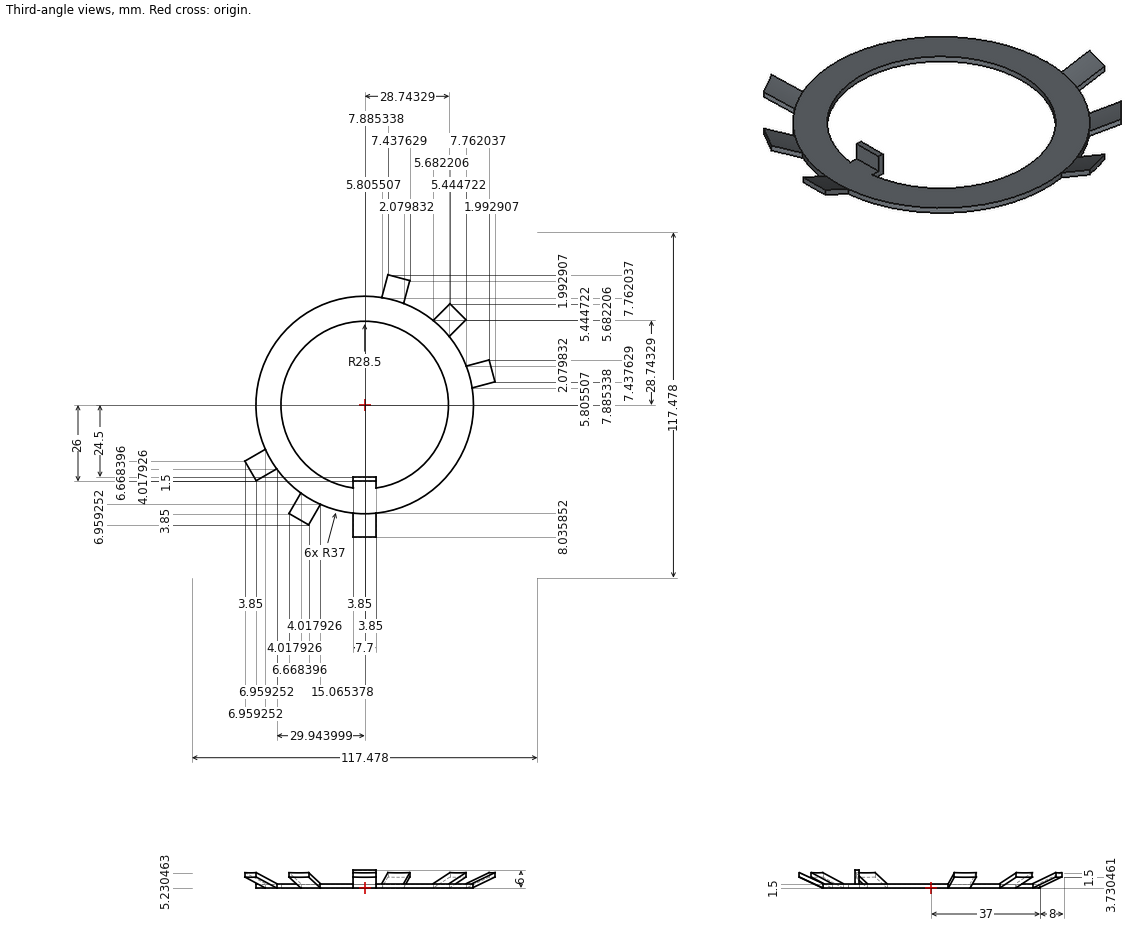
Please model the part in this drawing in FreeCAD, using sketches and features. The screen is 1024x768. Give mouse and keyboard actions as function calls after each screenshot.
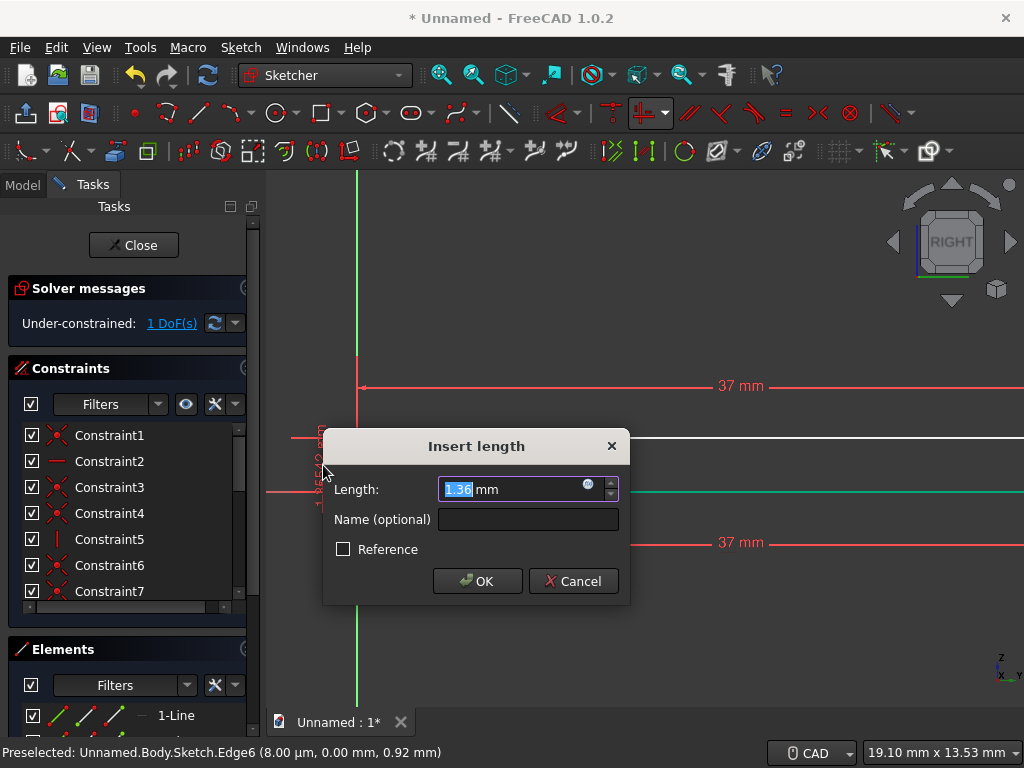
text(1.5)
key(Return)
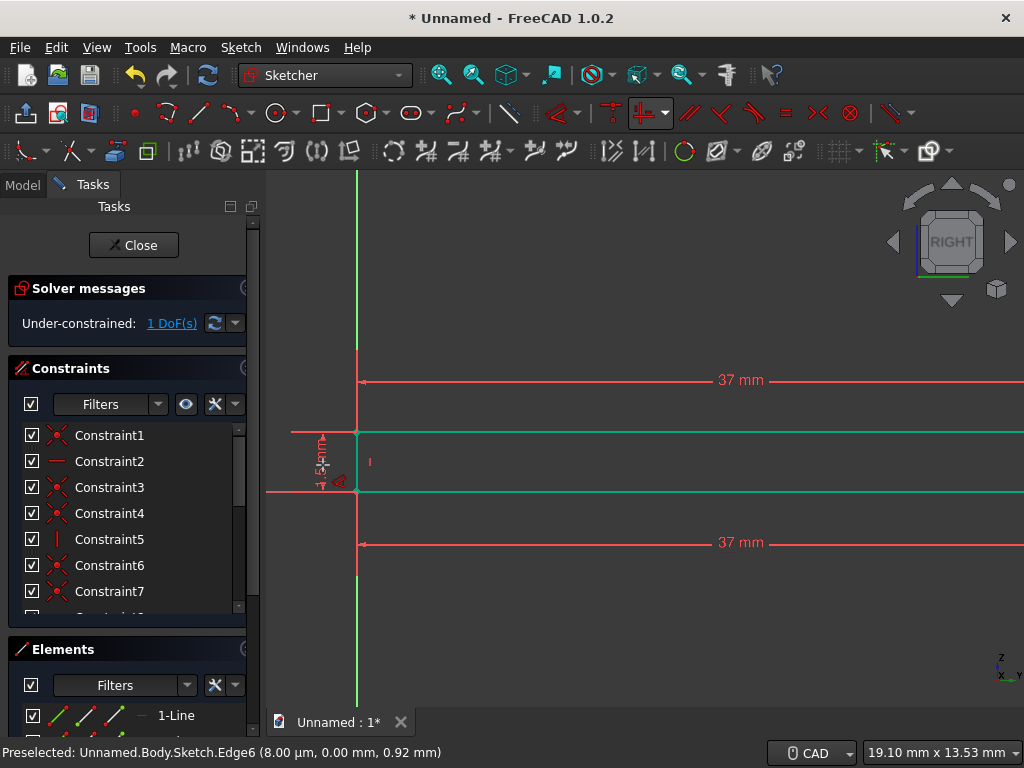
scroll(356, 455, down, 7)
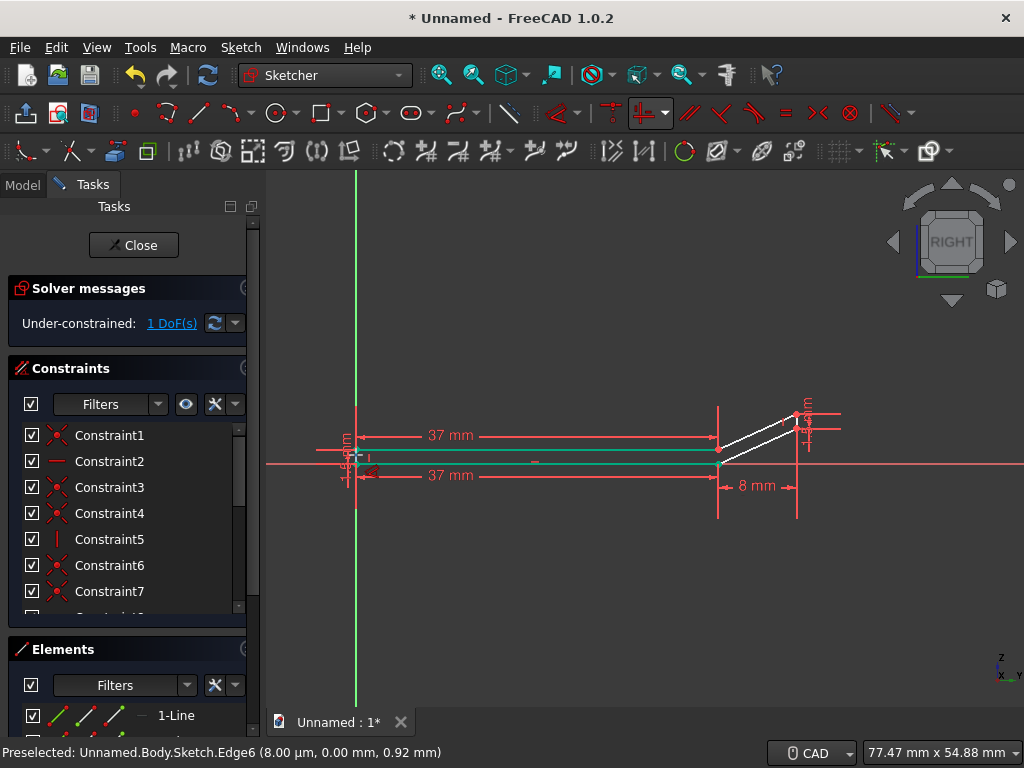
click(797, 429)
click(831, 447)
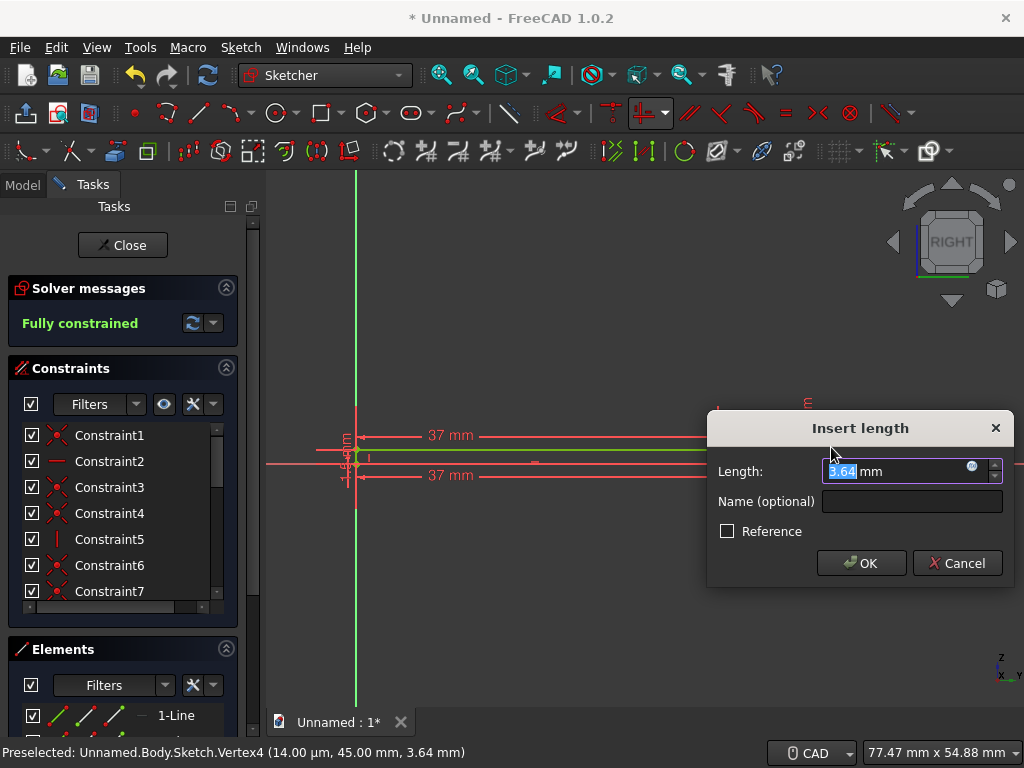
text(3.730461)
key(Return)
key(Escape)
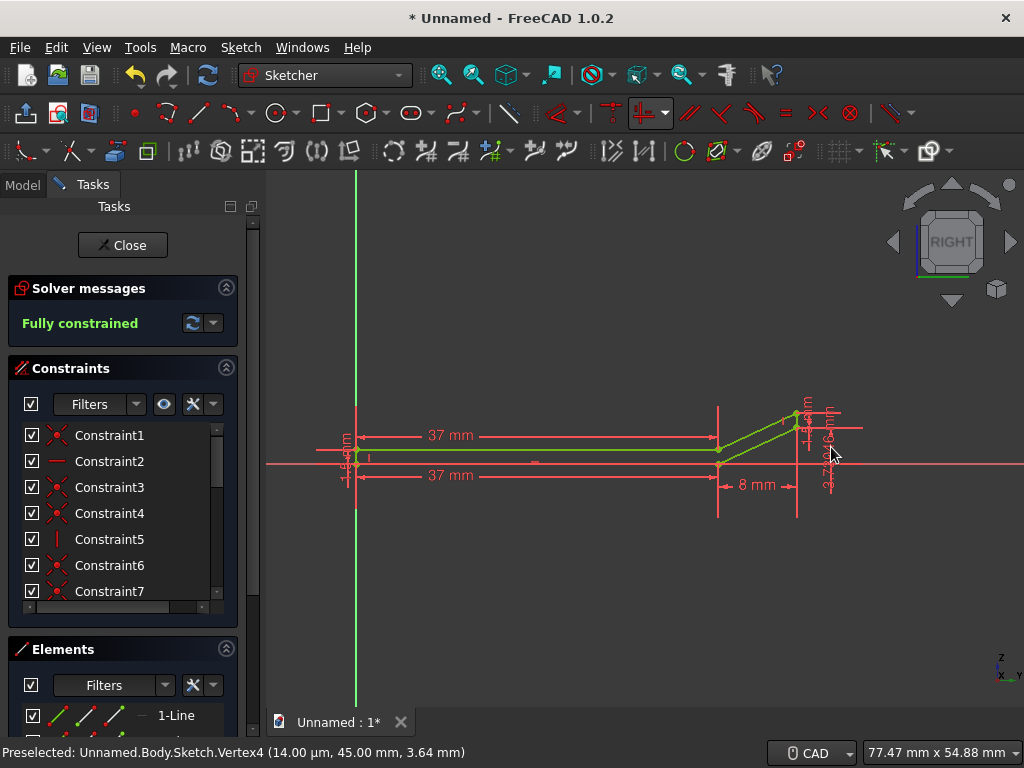
click(123, 245)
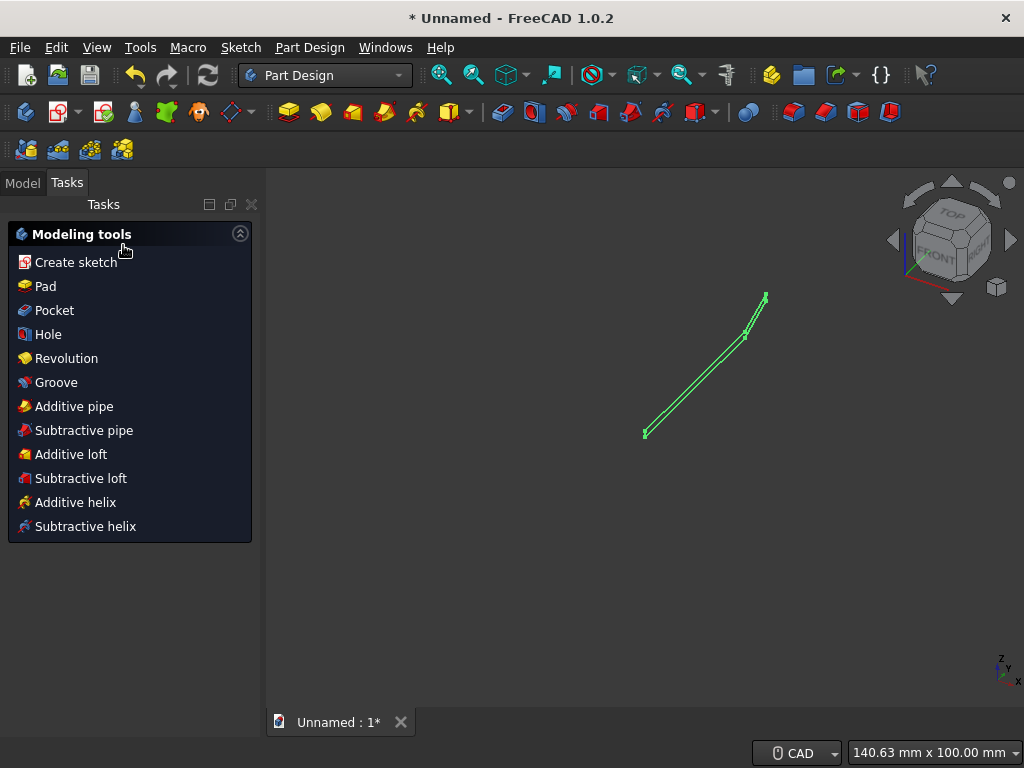
click(322, 112)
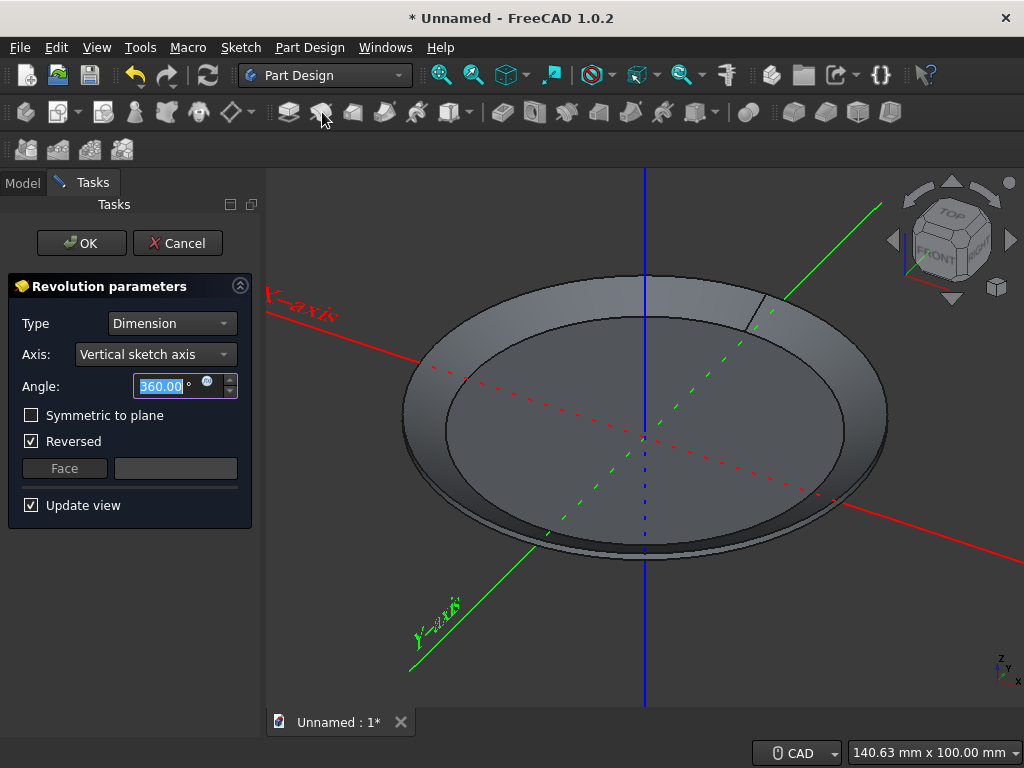
click(82, 243)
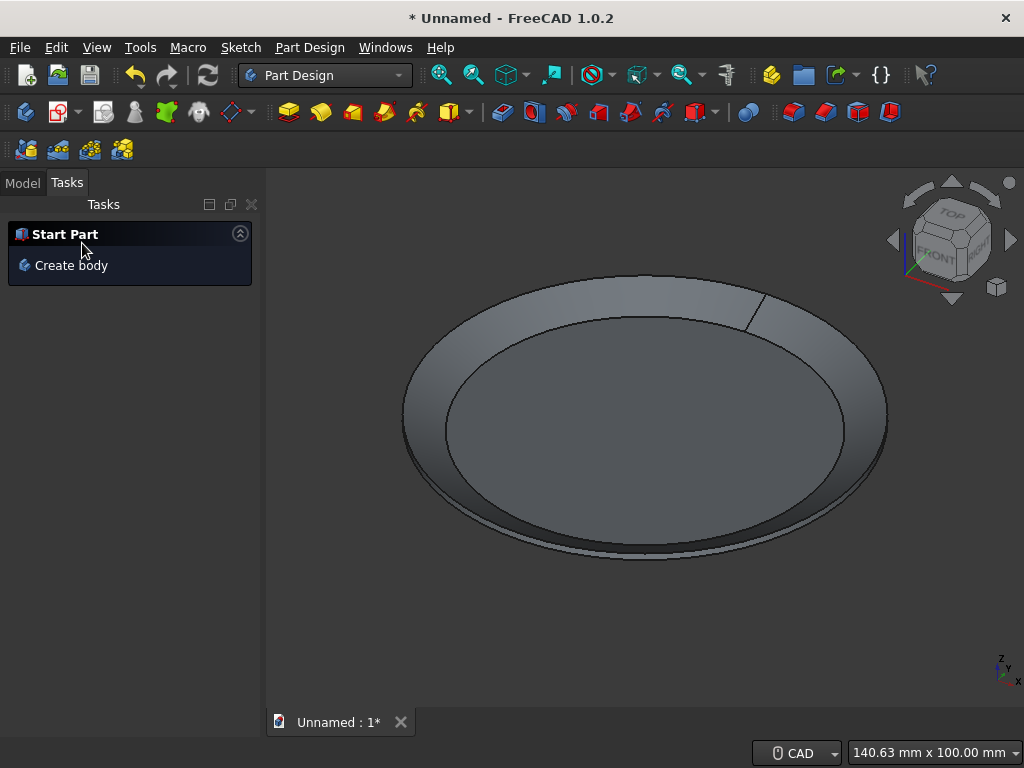
click(58, 112)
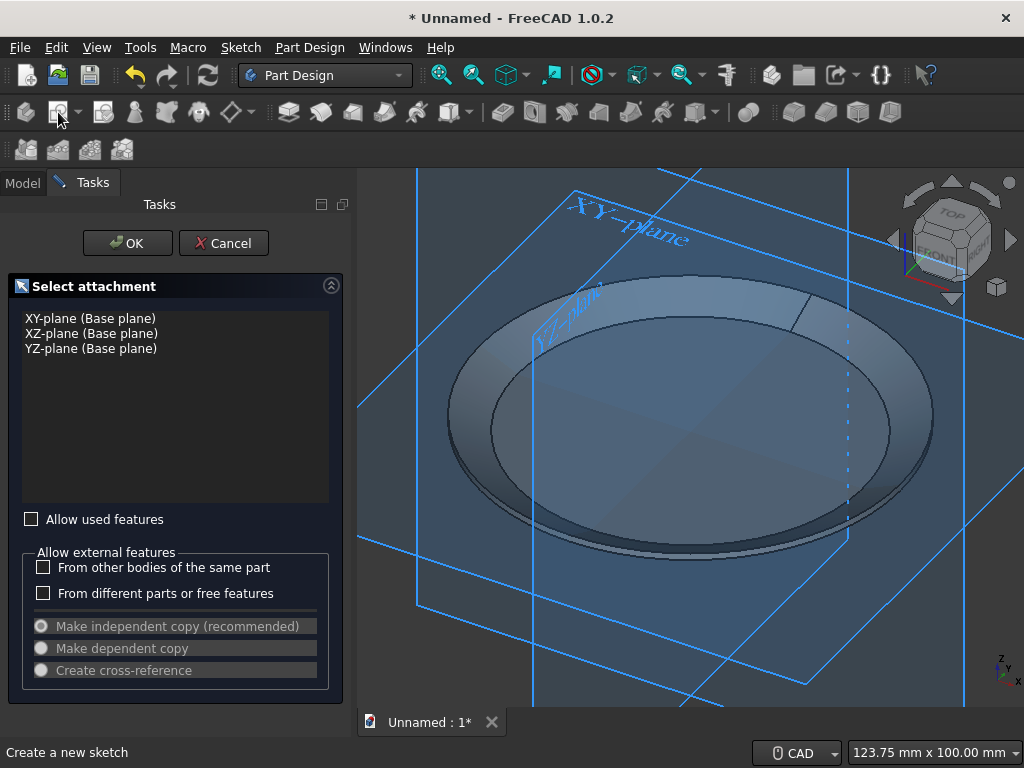
click(82, 318)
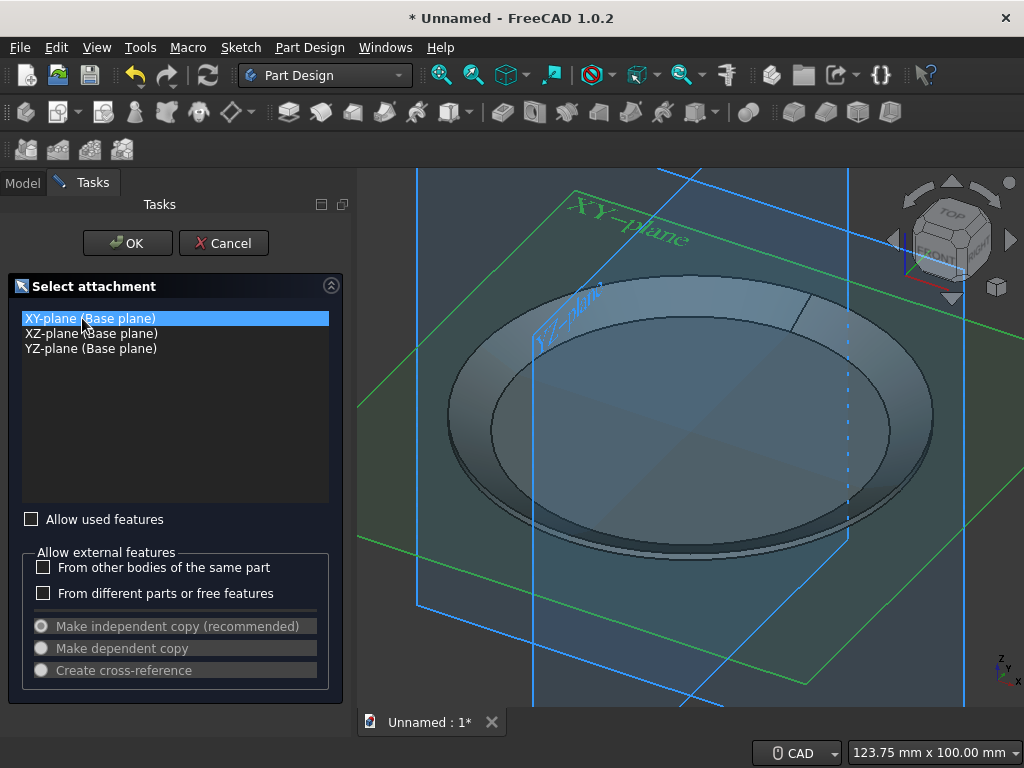
click(128, 243)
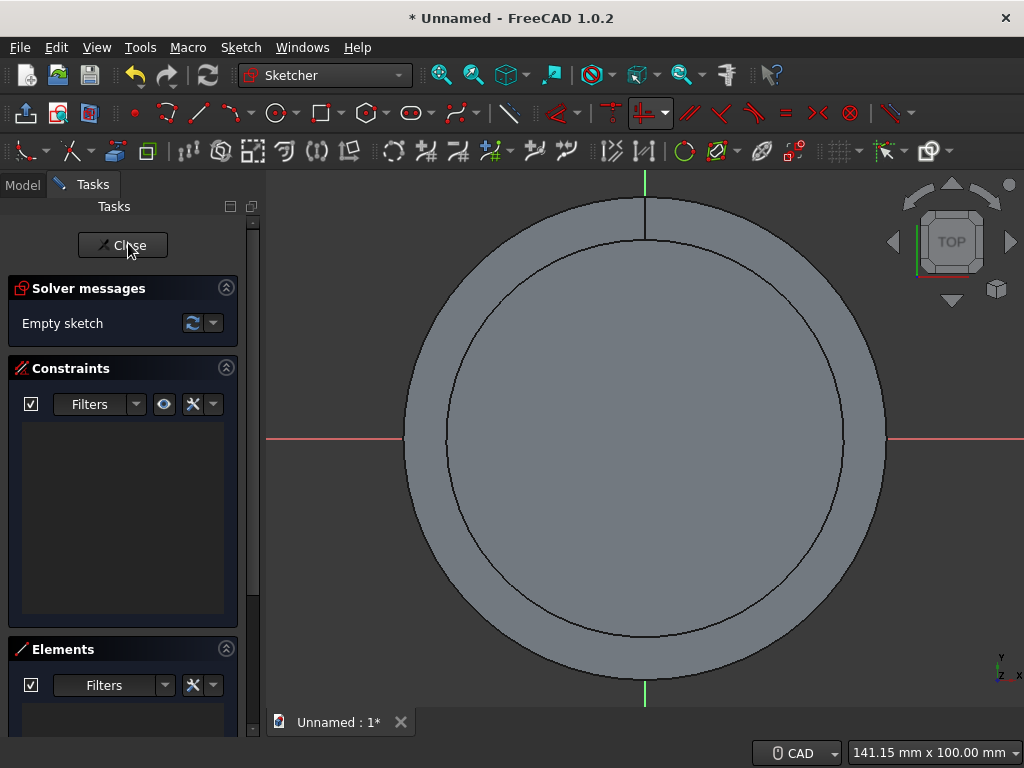
click(90, 114)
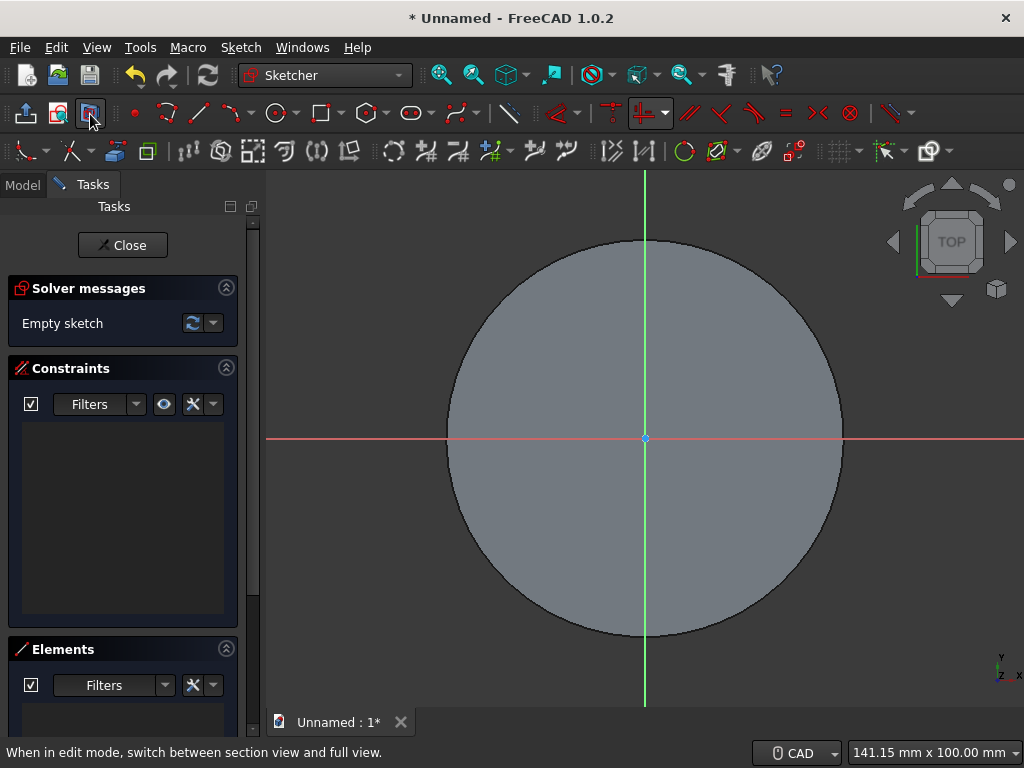
scroll(493, 439, down, 3)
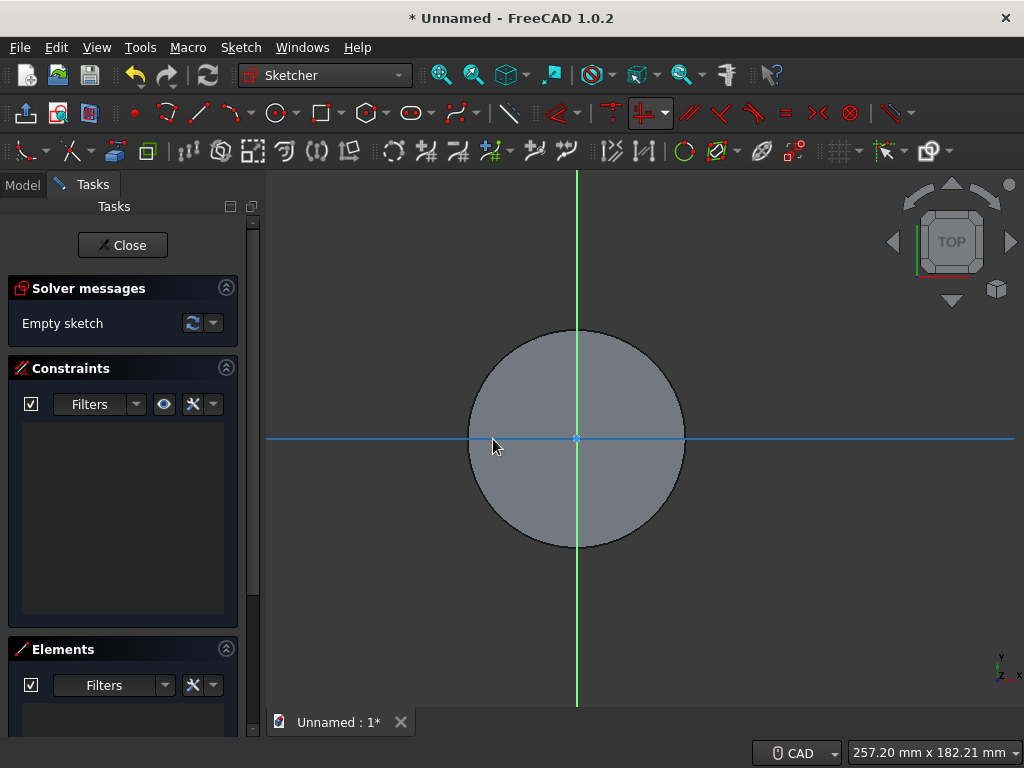
click(344, 114)